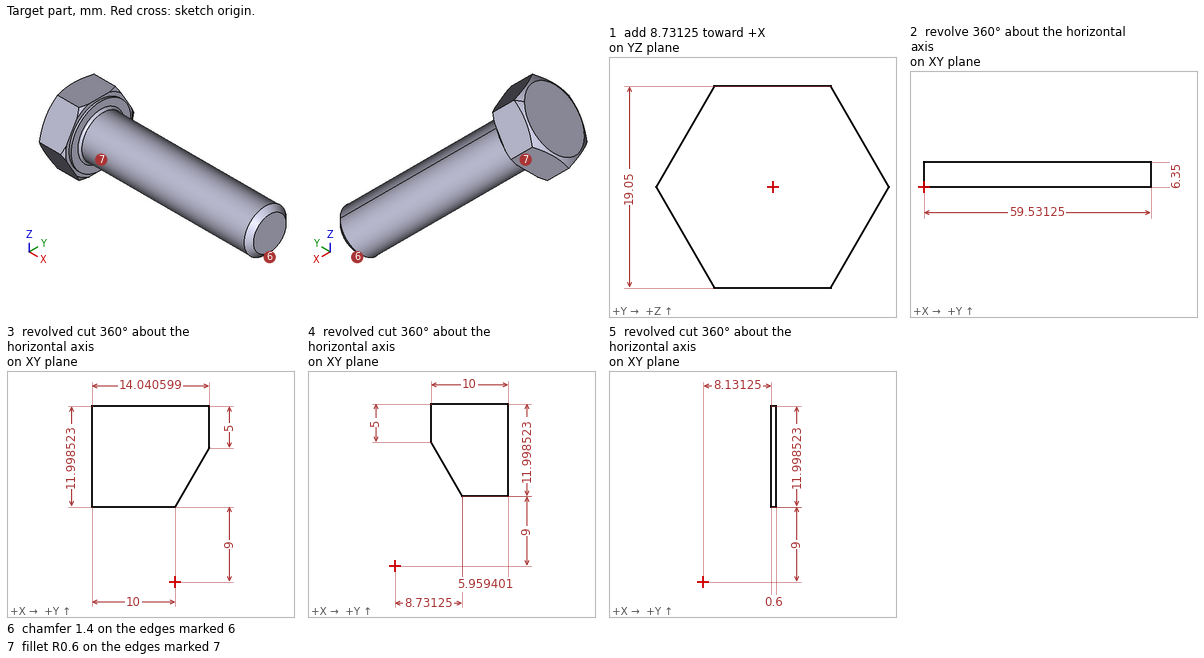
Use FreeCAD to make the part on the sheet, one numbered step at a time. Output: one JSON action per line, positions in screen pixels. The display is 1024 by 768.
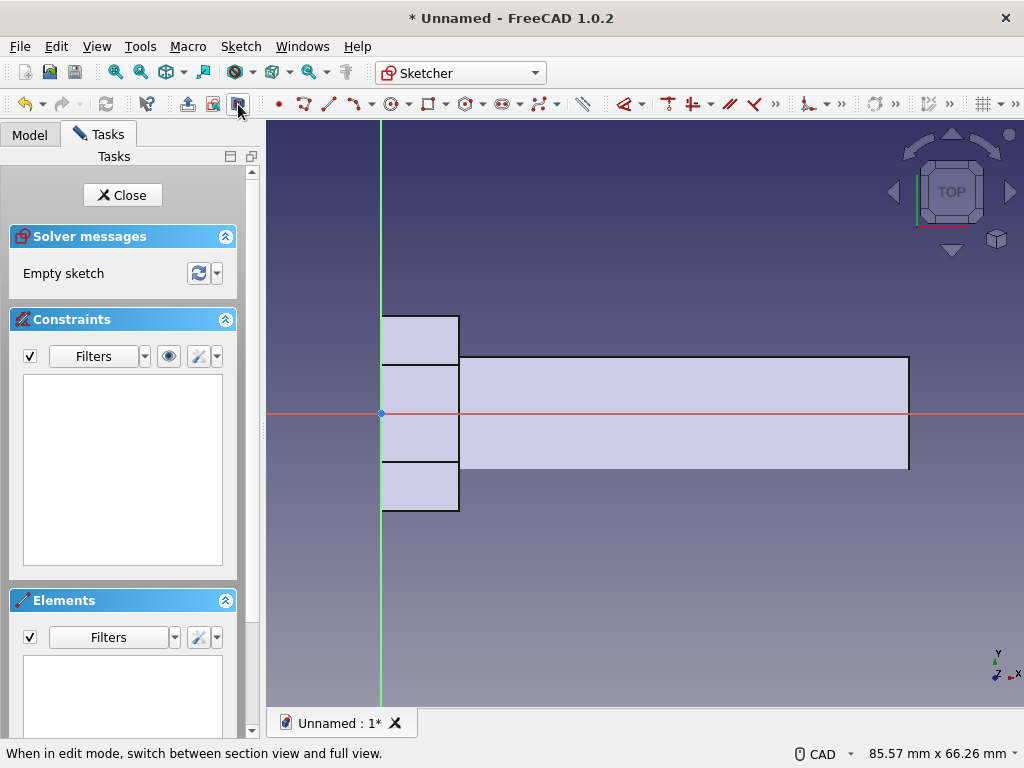
{"action": "scroll", "coordinate": [576, 414], "scroll_direction": "down", "scroll_amount": 5}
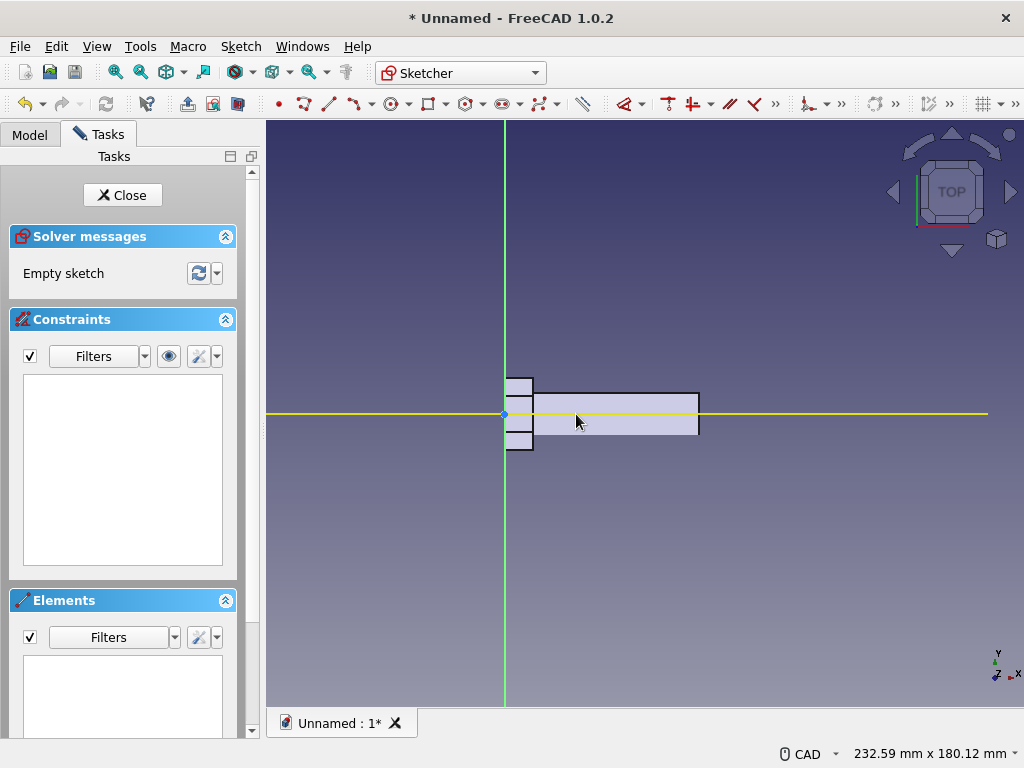
{"action": "scroll", "coordinate": [479, 373], "scroll_direction": "up", "scroll_amount": 9}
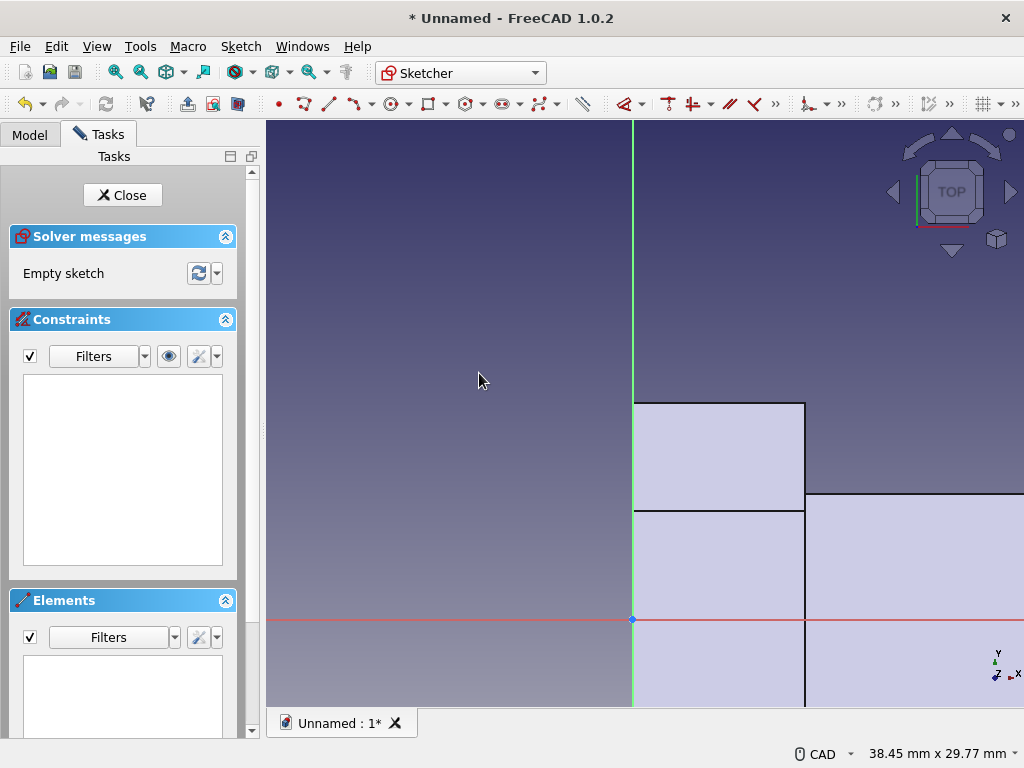
{"action": "left_click", "coordinate": [304, 104]}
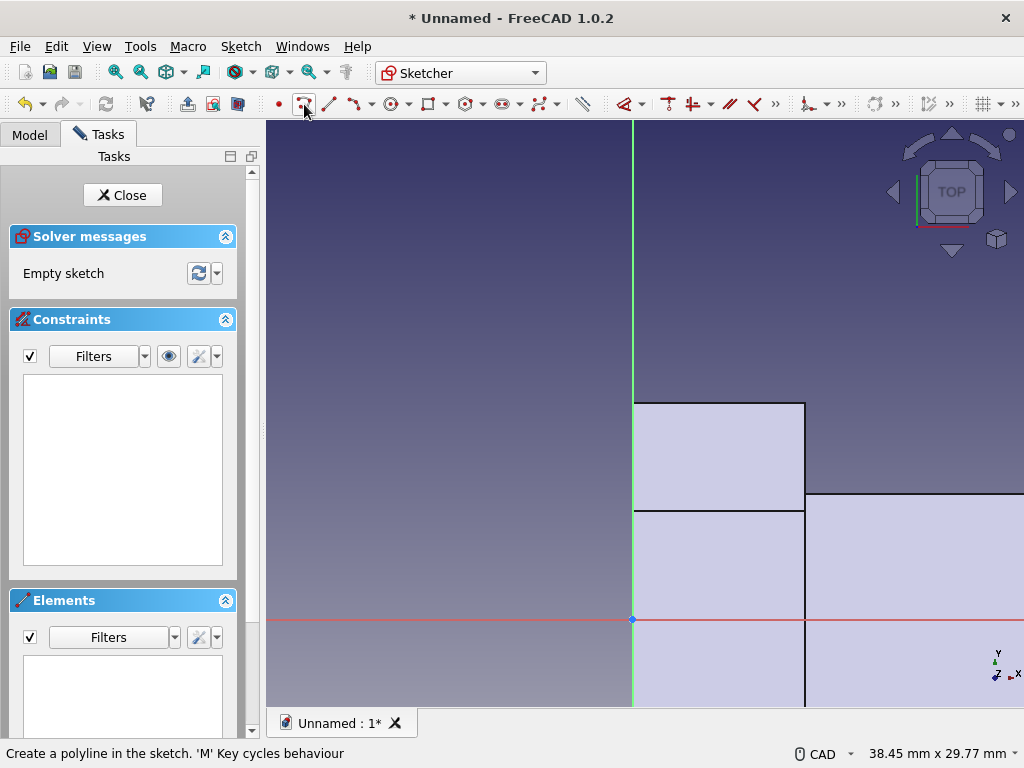
{"action": "left_click", "coordinate": [633, 442]}
{"action": "left_click", "coordinate": [712, 304]}
{"action": "left_click", "coordinate": [712, 206]}
{"action": "left_click", "coordinate": [436, 206]}
{"action": "left_click", "coordinate": [436, 442]}
{"action": "left_click", "coordinate": [633, 443]}
{"action": "key", "text": "Escape"}
{"action": "key", "text": "Escape"}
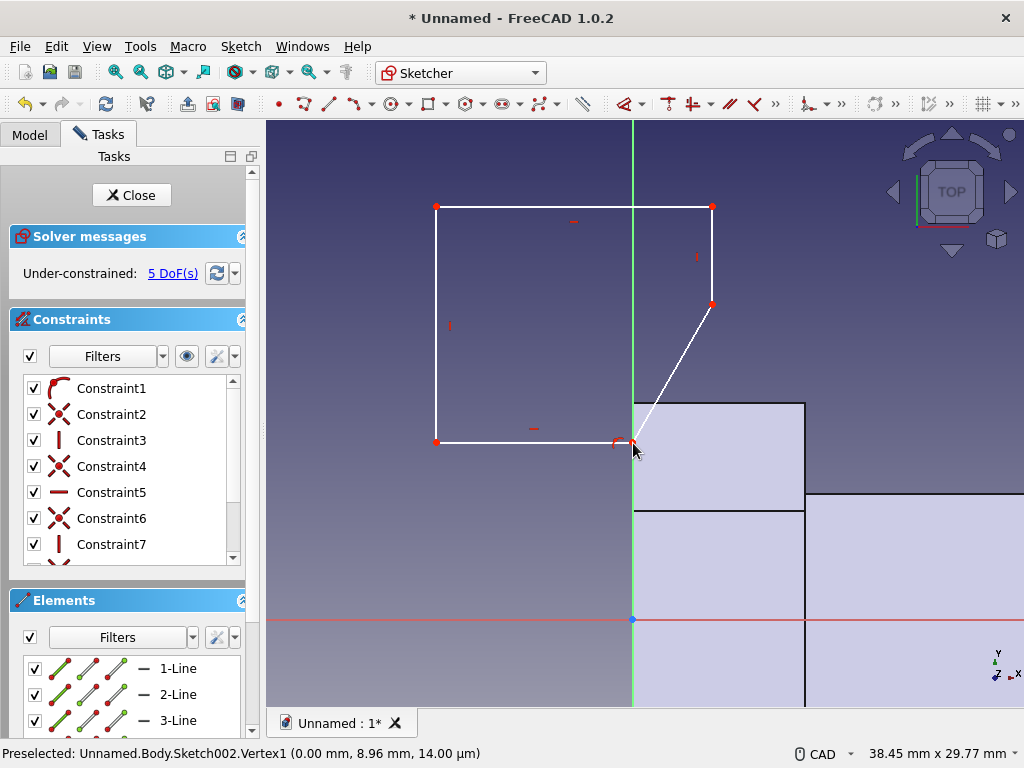
{"action": "left_click", "coordinate": [624, 104]}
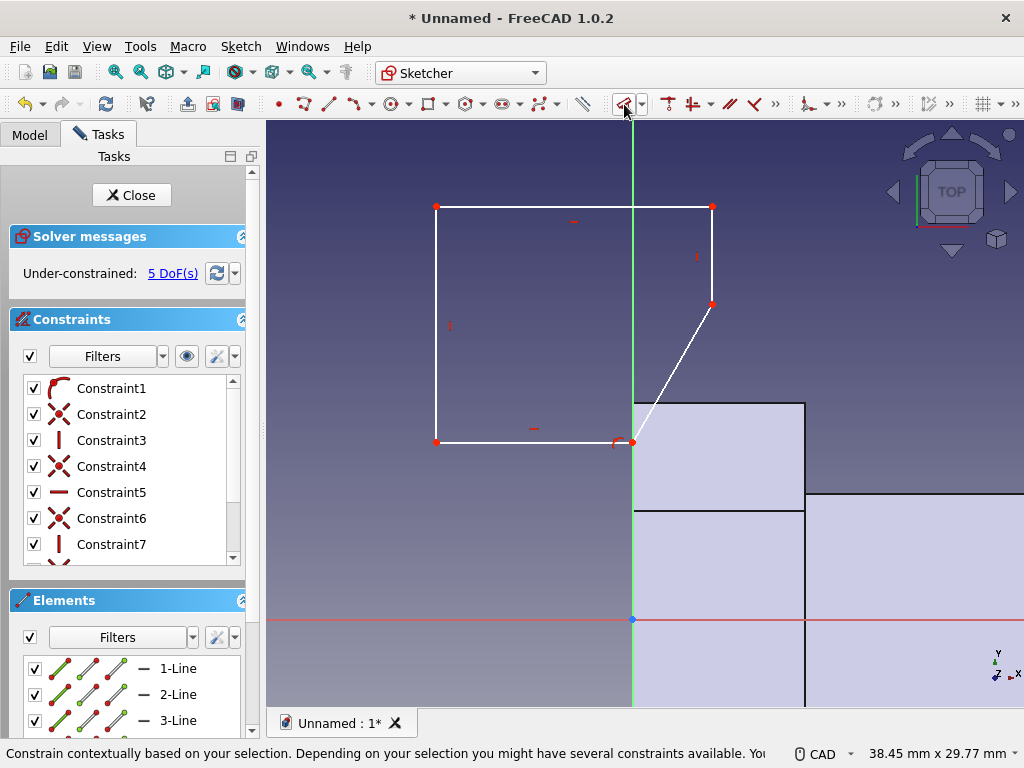
{"action": "left_click", "coordinate": [712, 276]}
{"action": "left_click", "coordinate": [746, 256]}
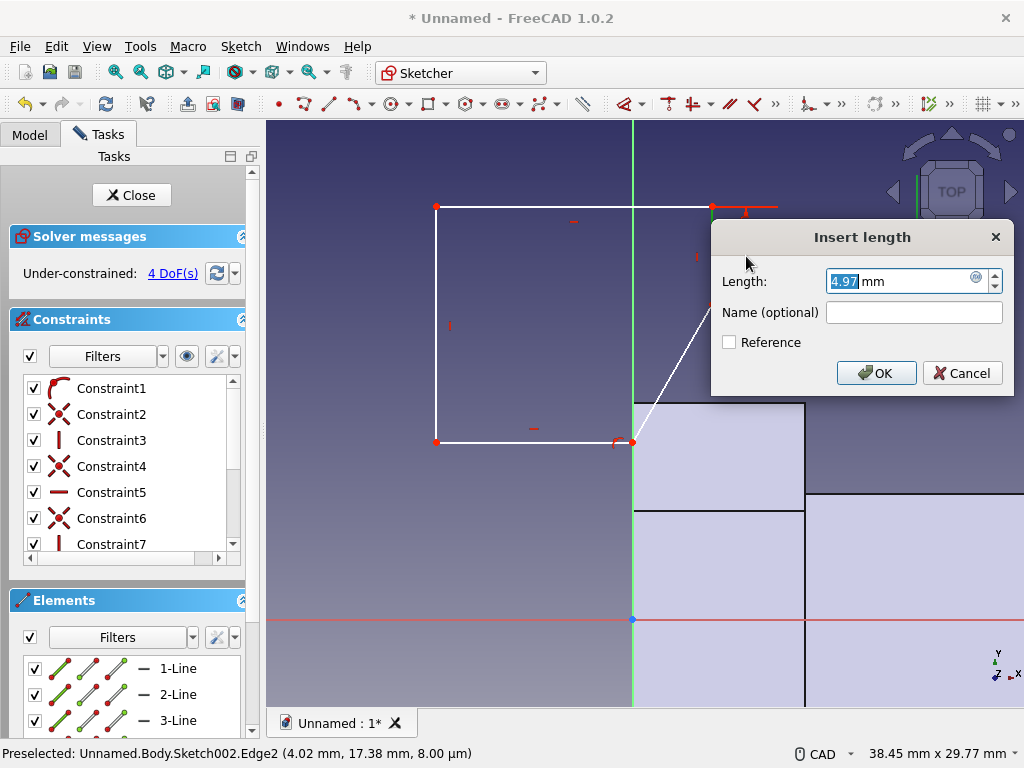
{"action": "type", "text": "5"}
{"action": "key", "text": "Return"}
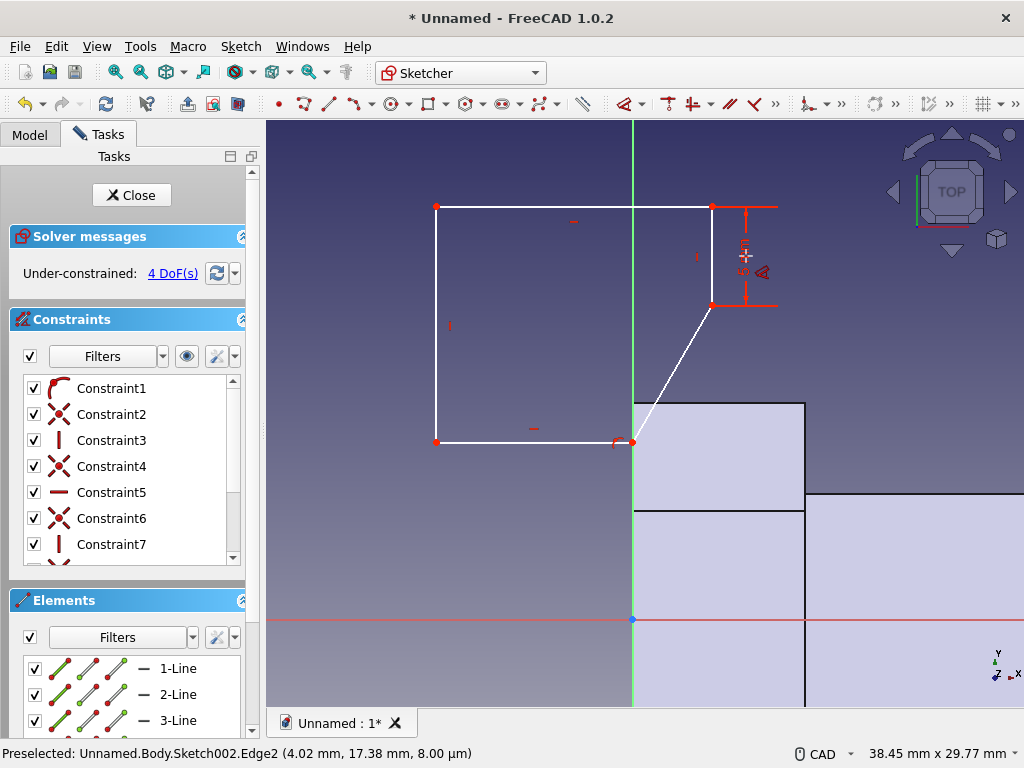
{"action": "left_click", "coordinate": [495, 443]}
{"action": "left_click", "coordinate": [534, 477]}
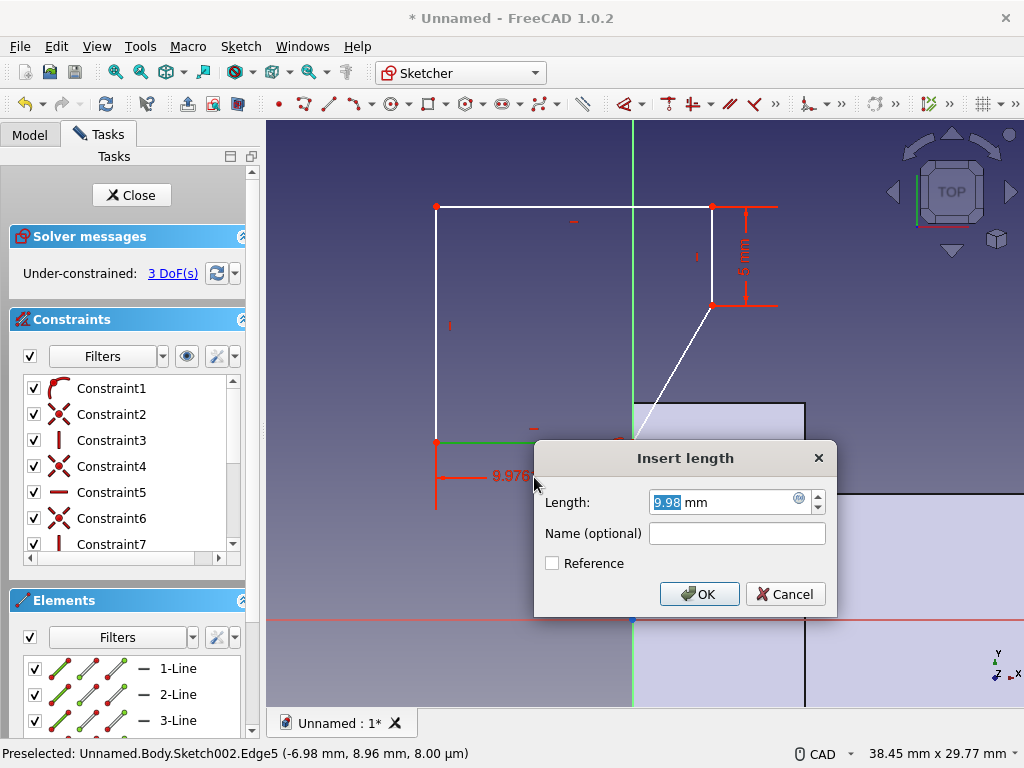
{"action": "type", "text": "10"}
{"action": "key", "text": "Return"}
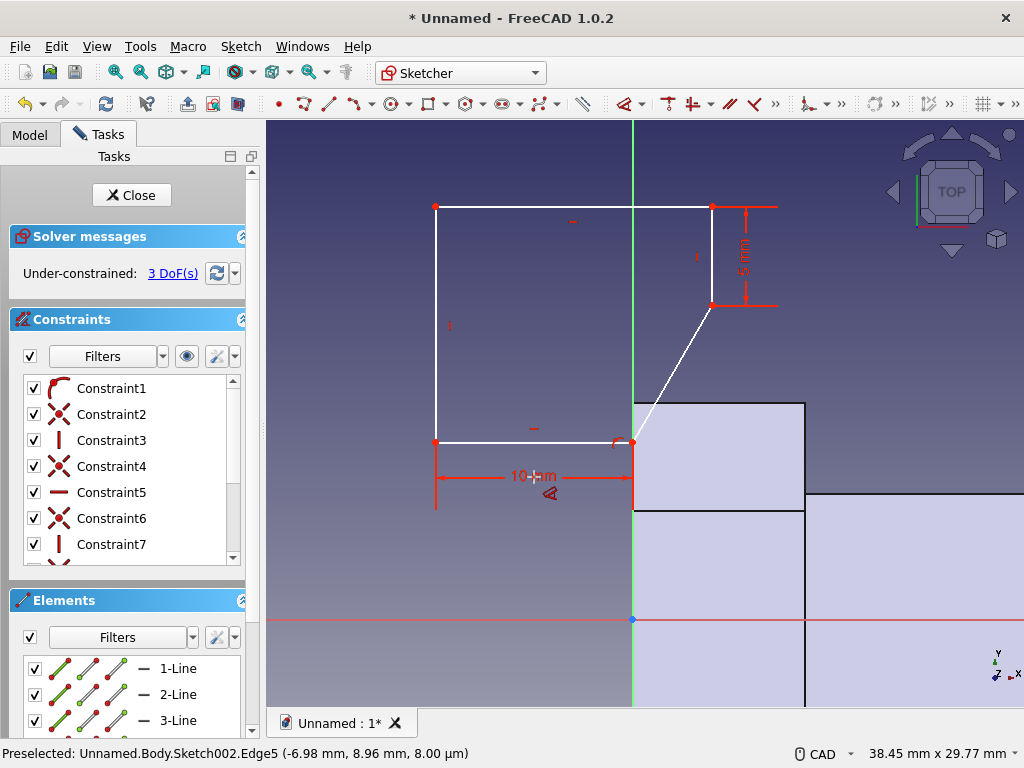
{"action": "left_click", "coordinate": [633, 443]}
{"action": "left_click", "coordinate": [667, 531]}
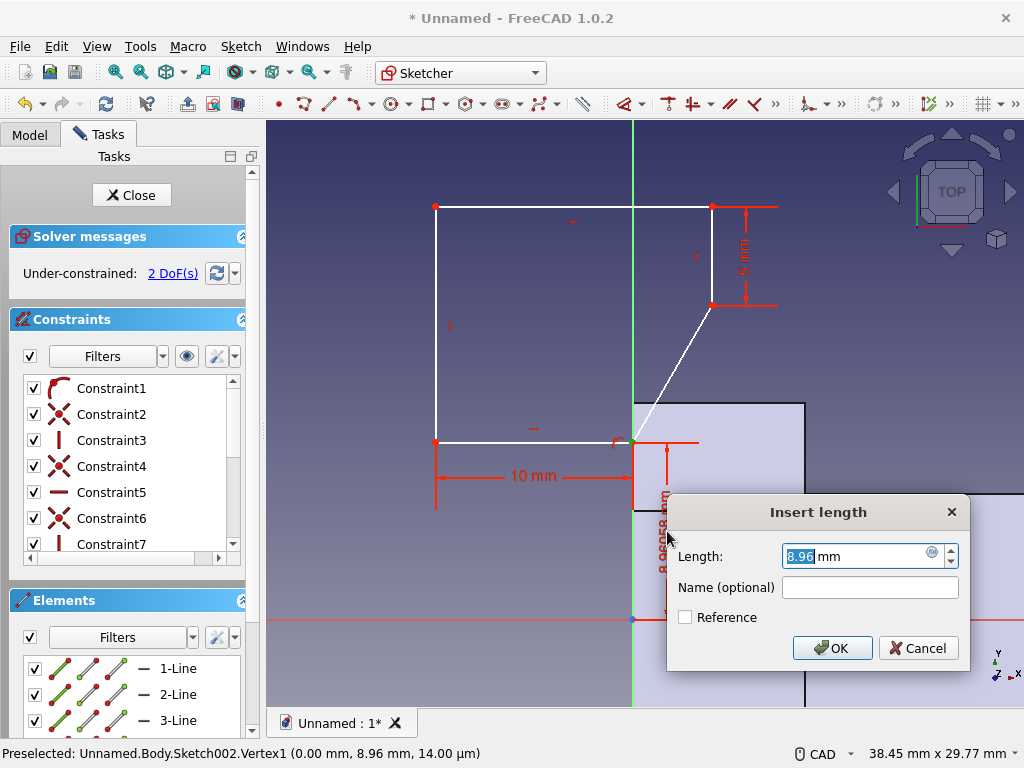
{"action": "type", "text": "9"}
{"action": "key", "text": "Return"}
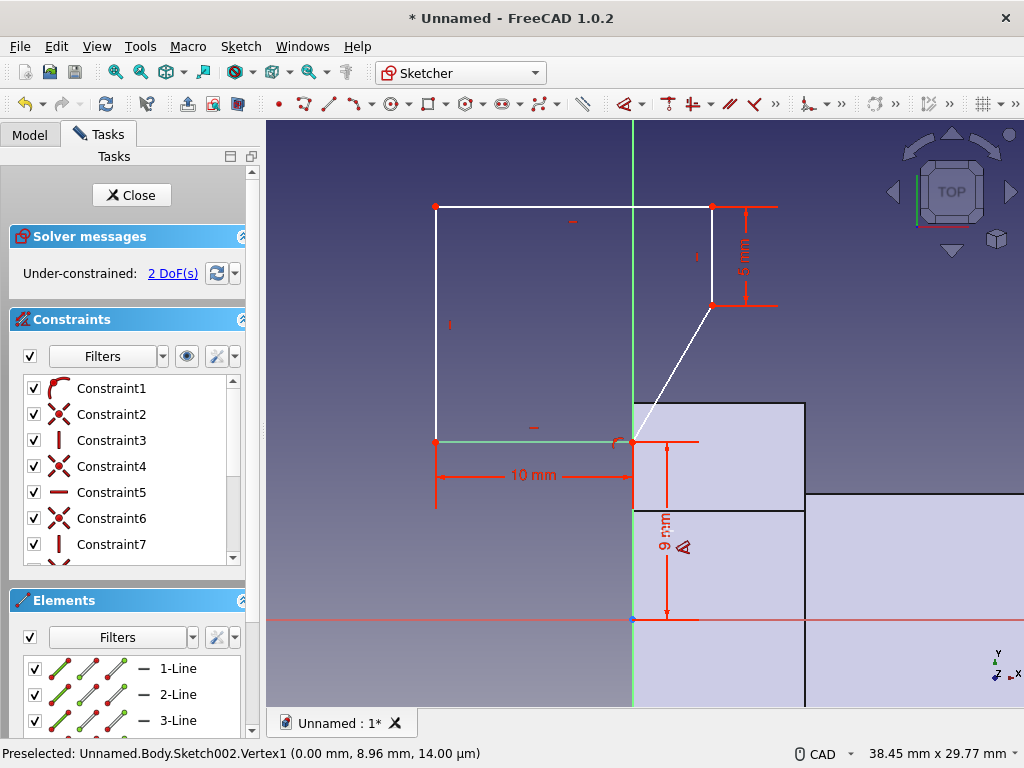
{"action": "left_click", "coordinate": [629, 207]}
{"action": "left_click", "coordinate": [574, 173]}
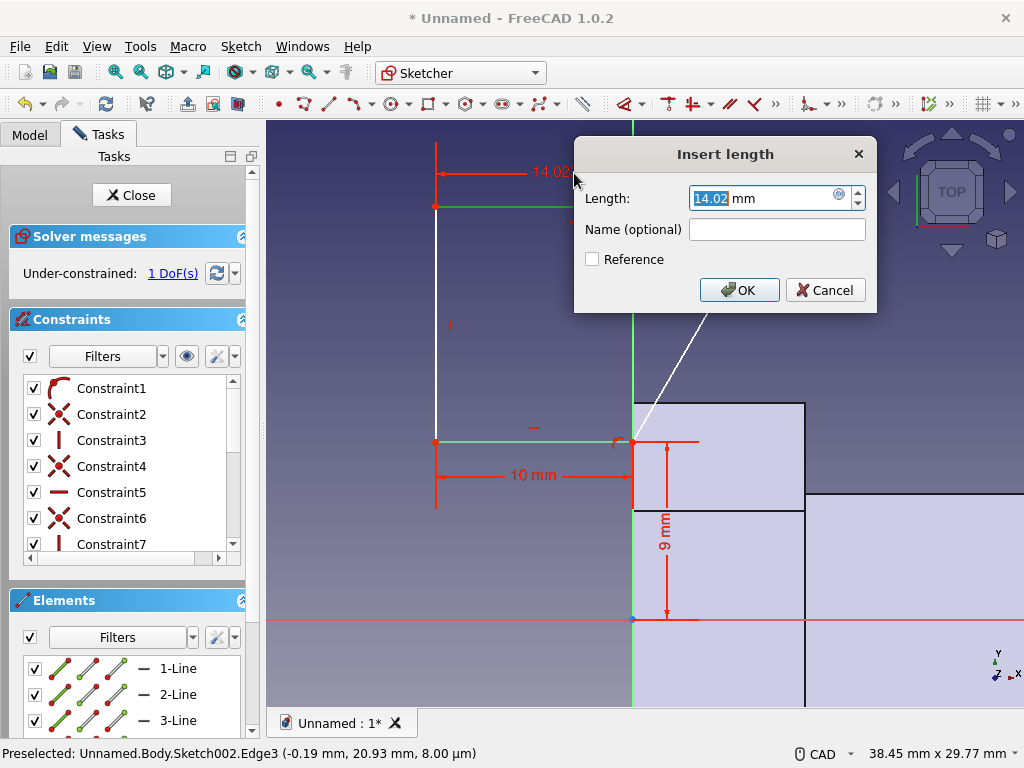
{"action": "type", "text": "14.040599"}
{"action": "key", "text": "Return"}